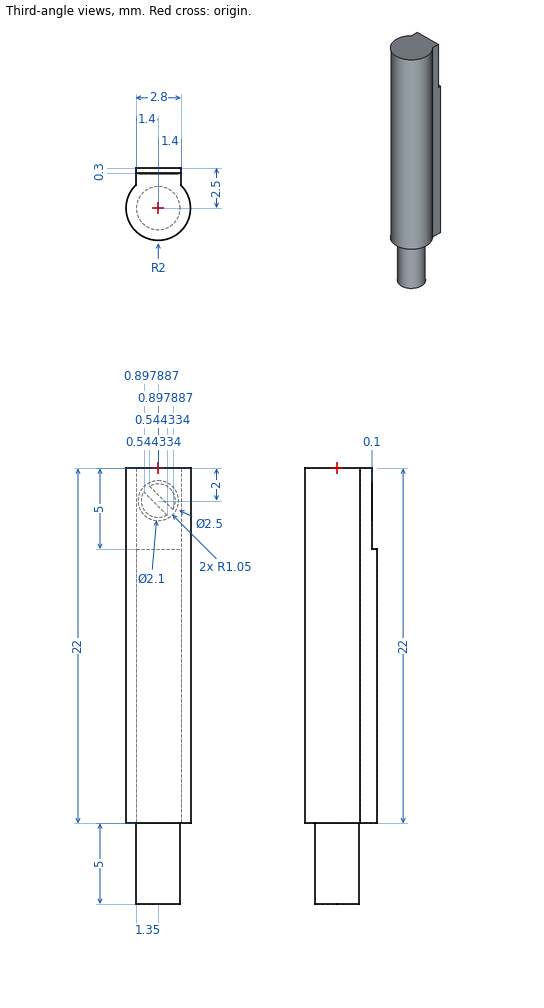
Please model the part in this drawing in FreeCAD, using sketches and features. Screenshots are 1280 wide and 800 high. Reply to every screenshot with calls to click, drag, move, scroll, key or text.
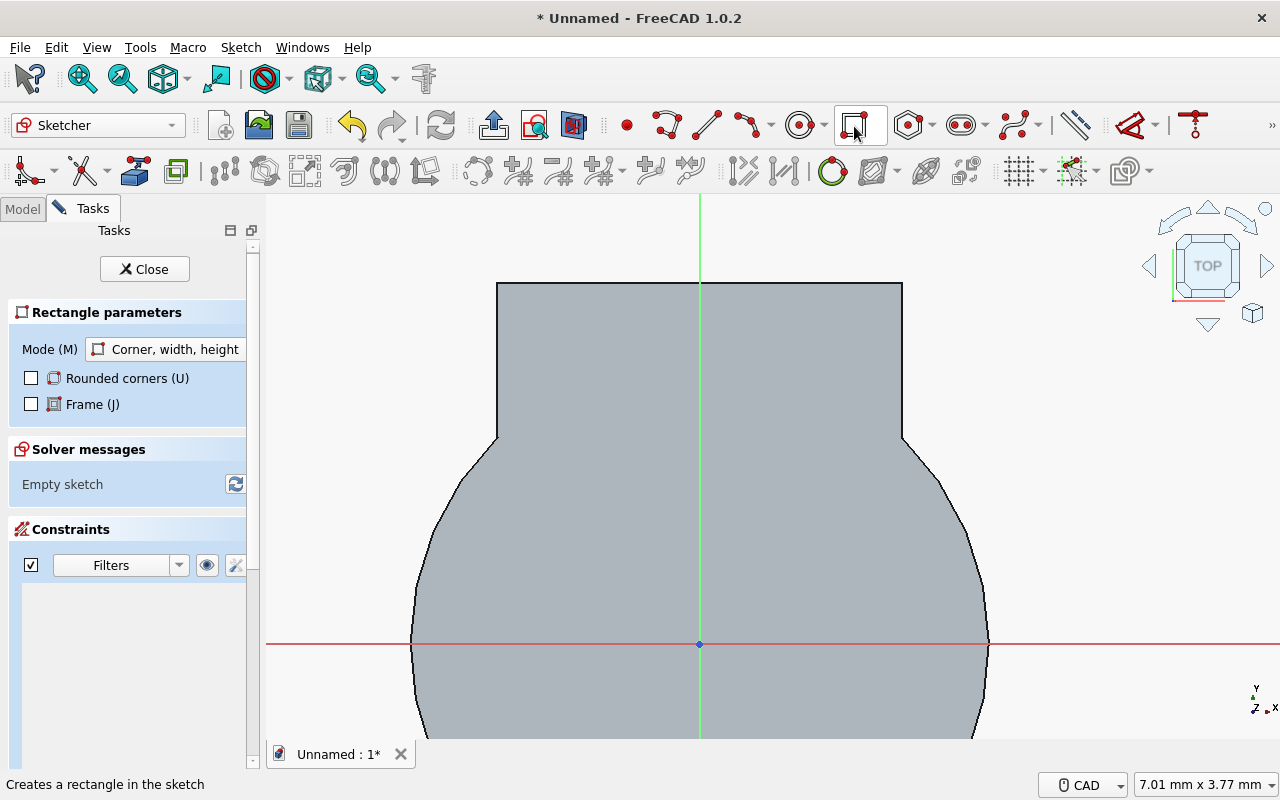
click(497, 283)
click(902, 326)
key(Escape)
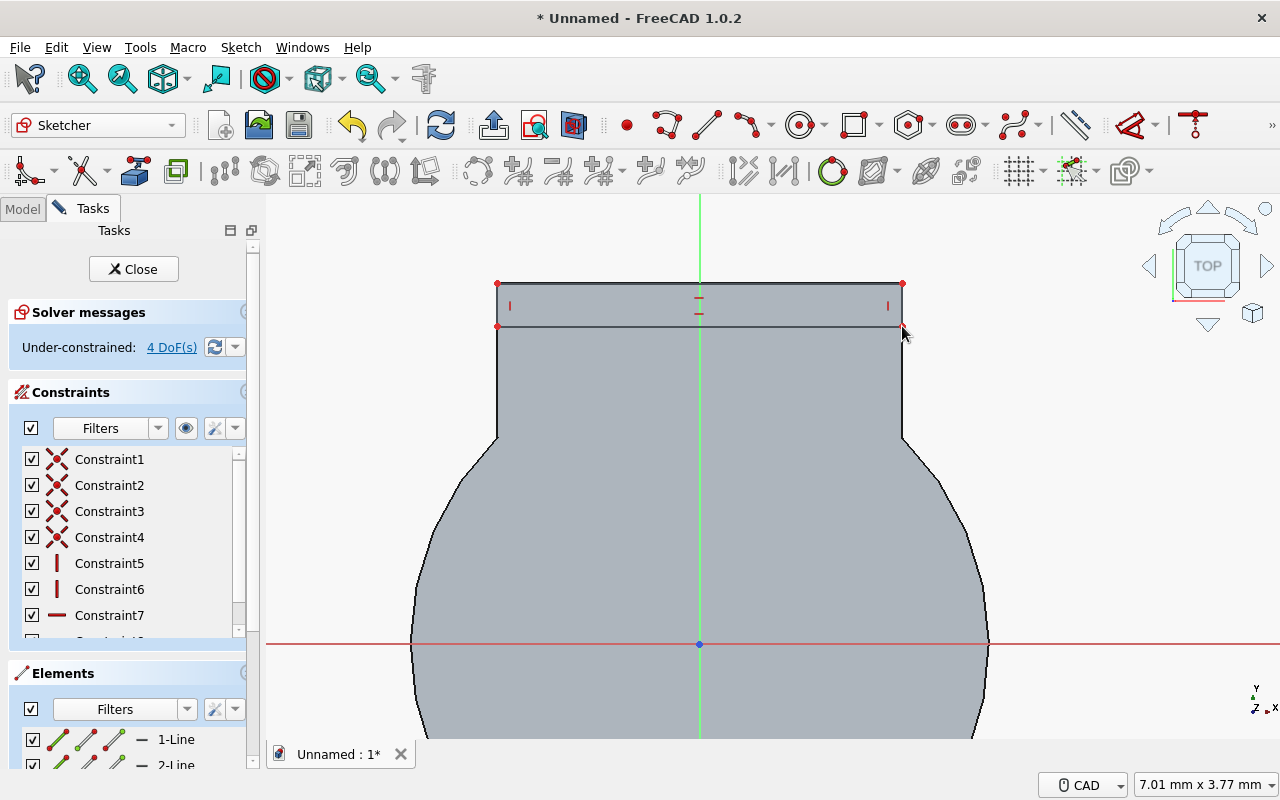
click(1130, 126)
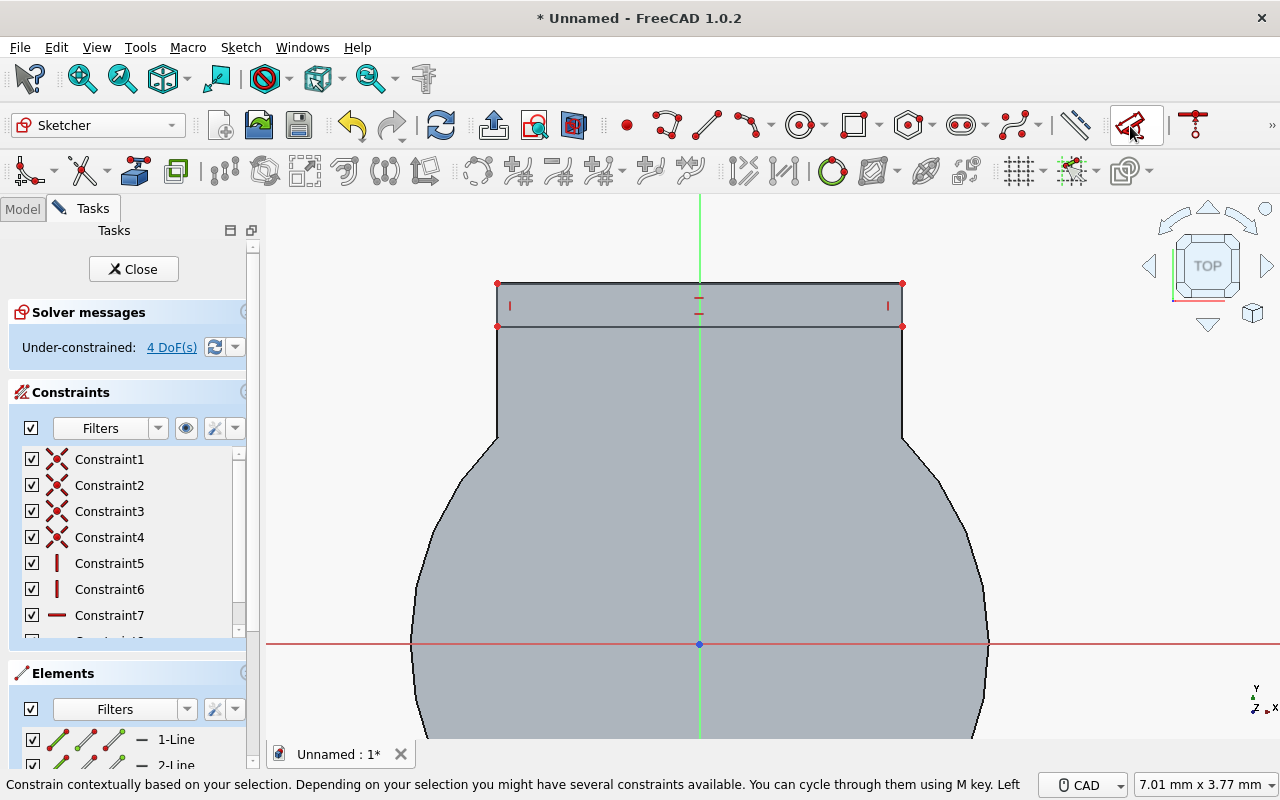
click(497, 297)
click(463, 305)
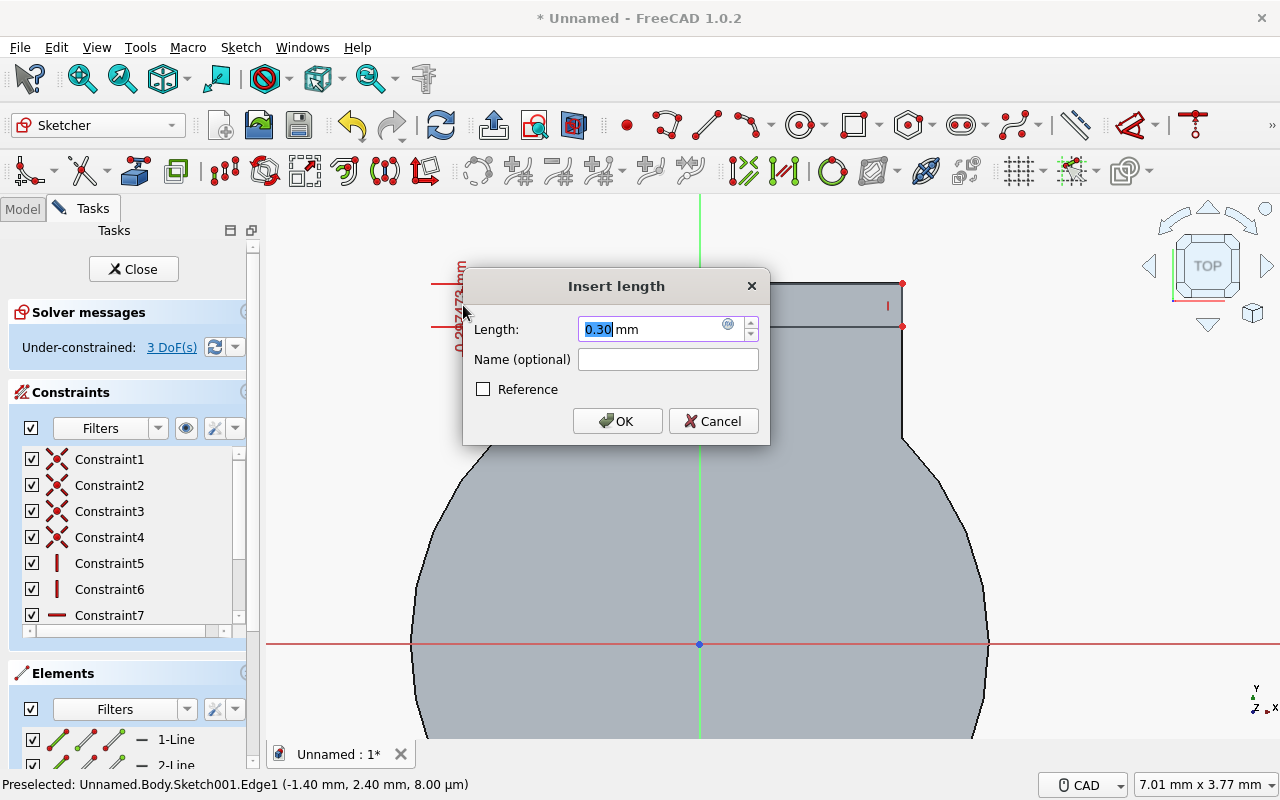
text(0.3)
key(Return)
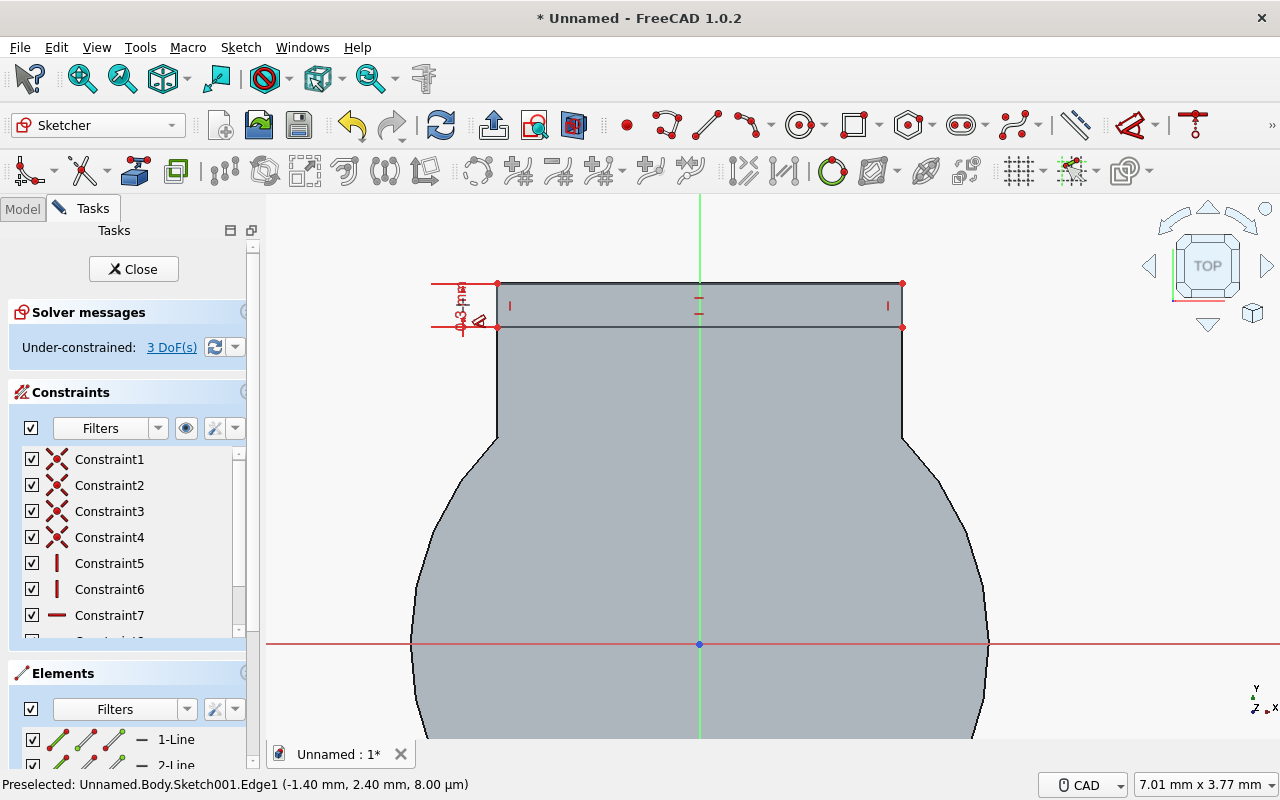
click(619, 327)
click(606, 361)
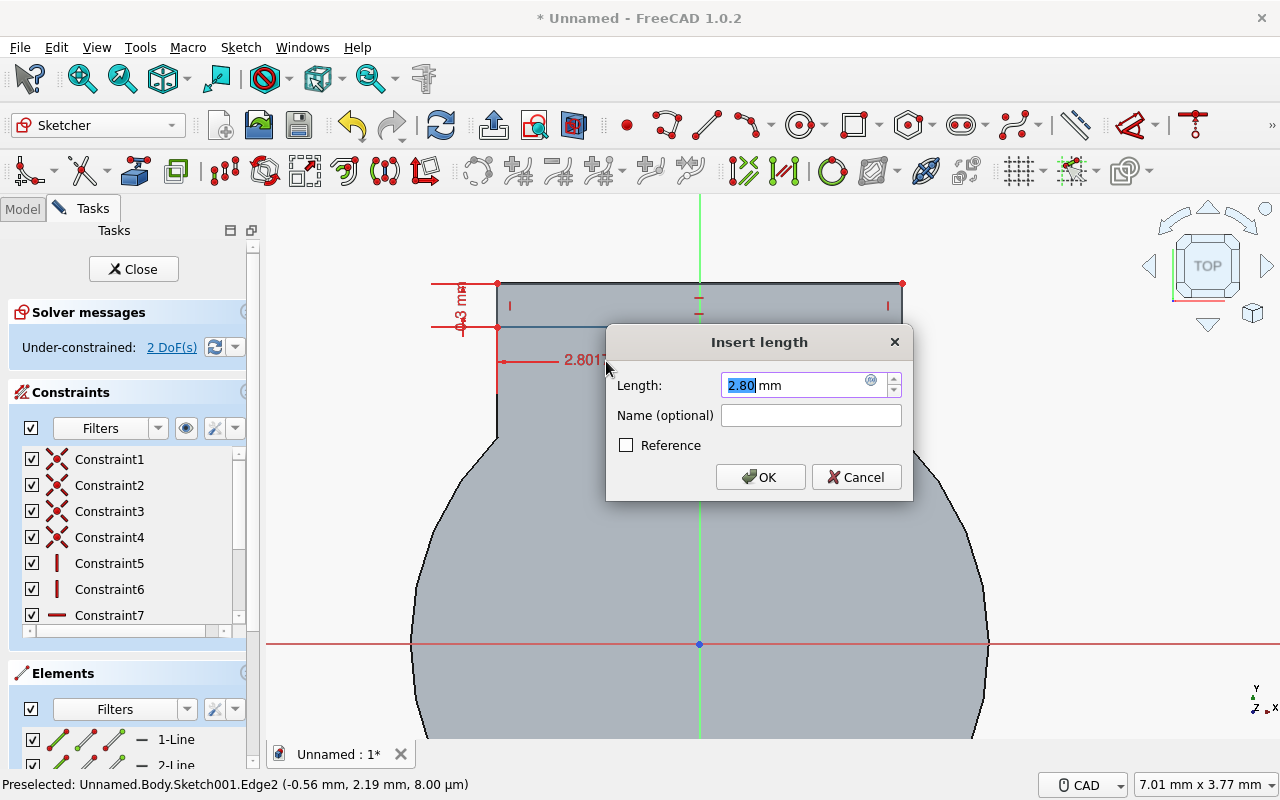
text(2.8)
key(Return)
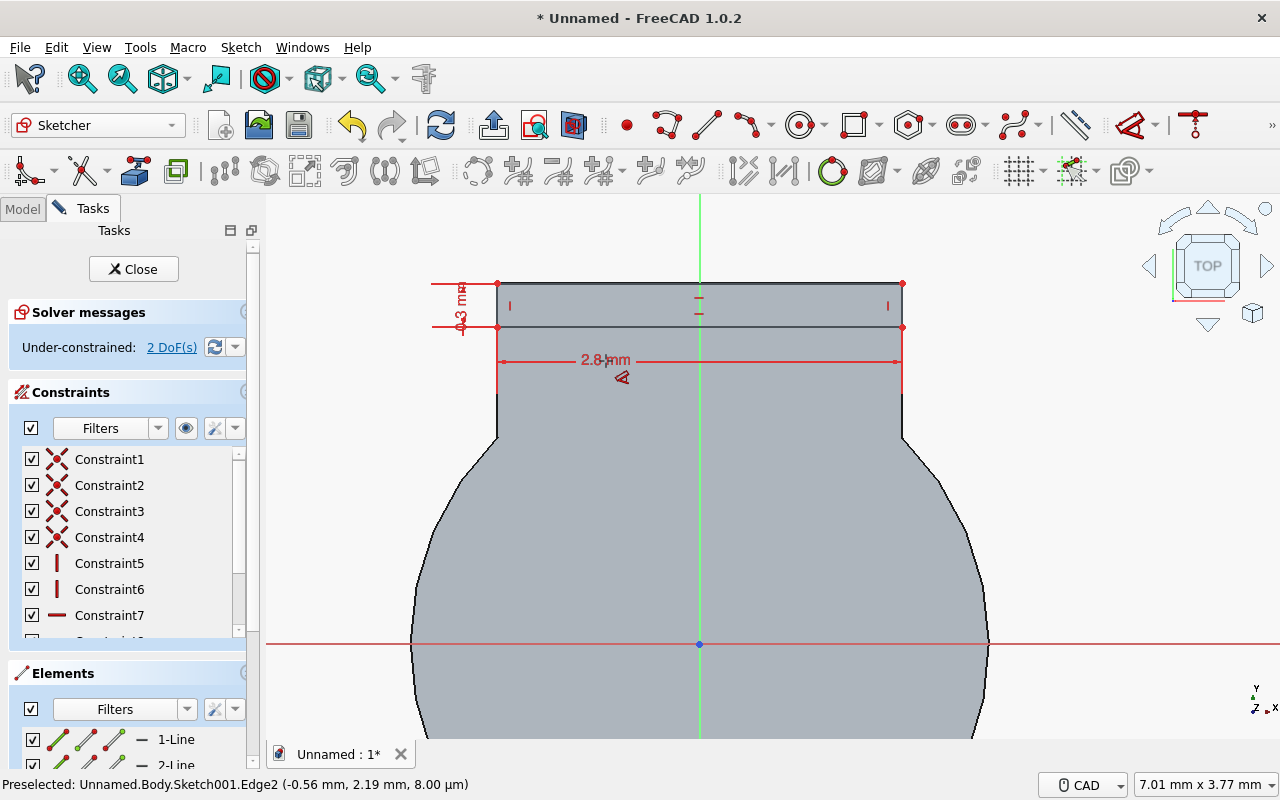
click(497, 284)
click(598, 678)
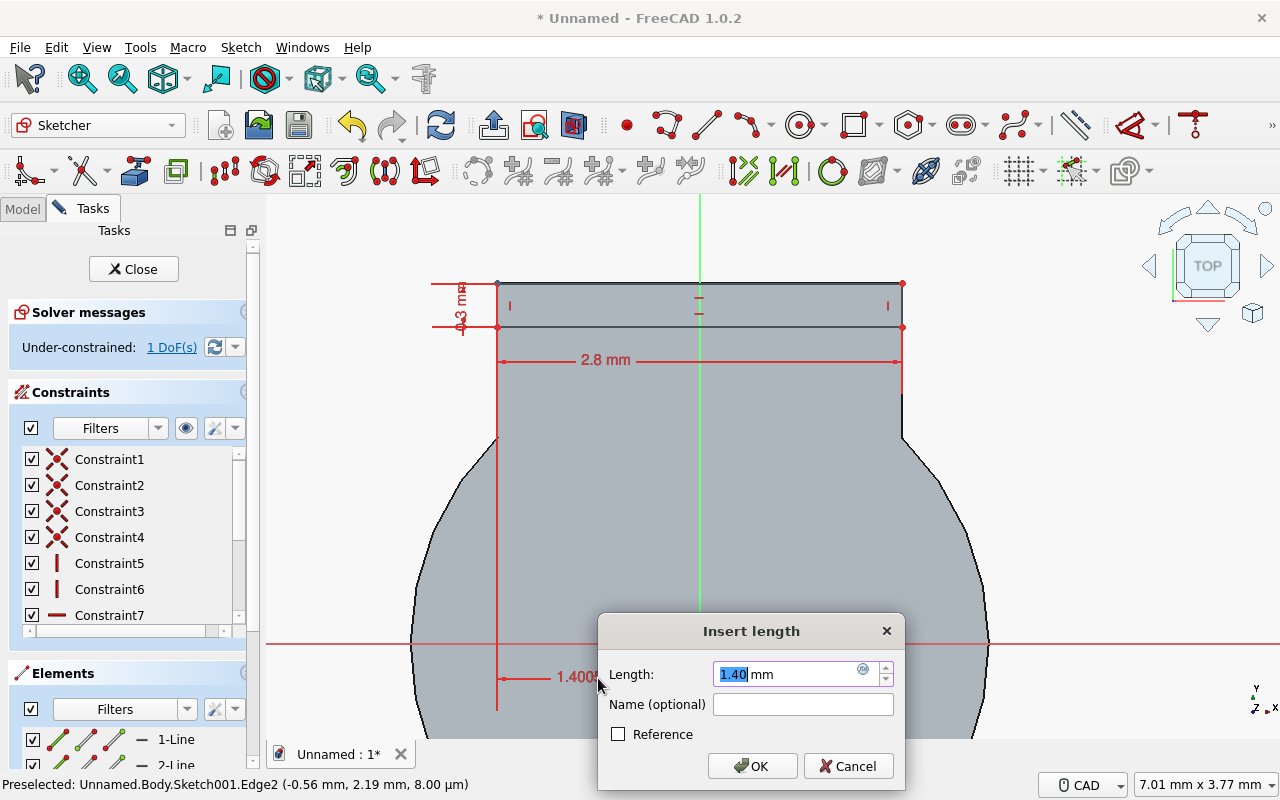
text(1.4)
key(Return)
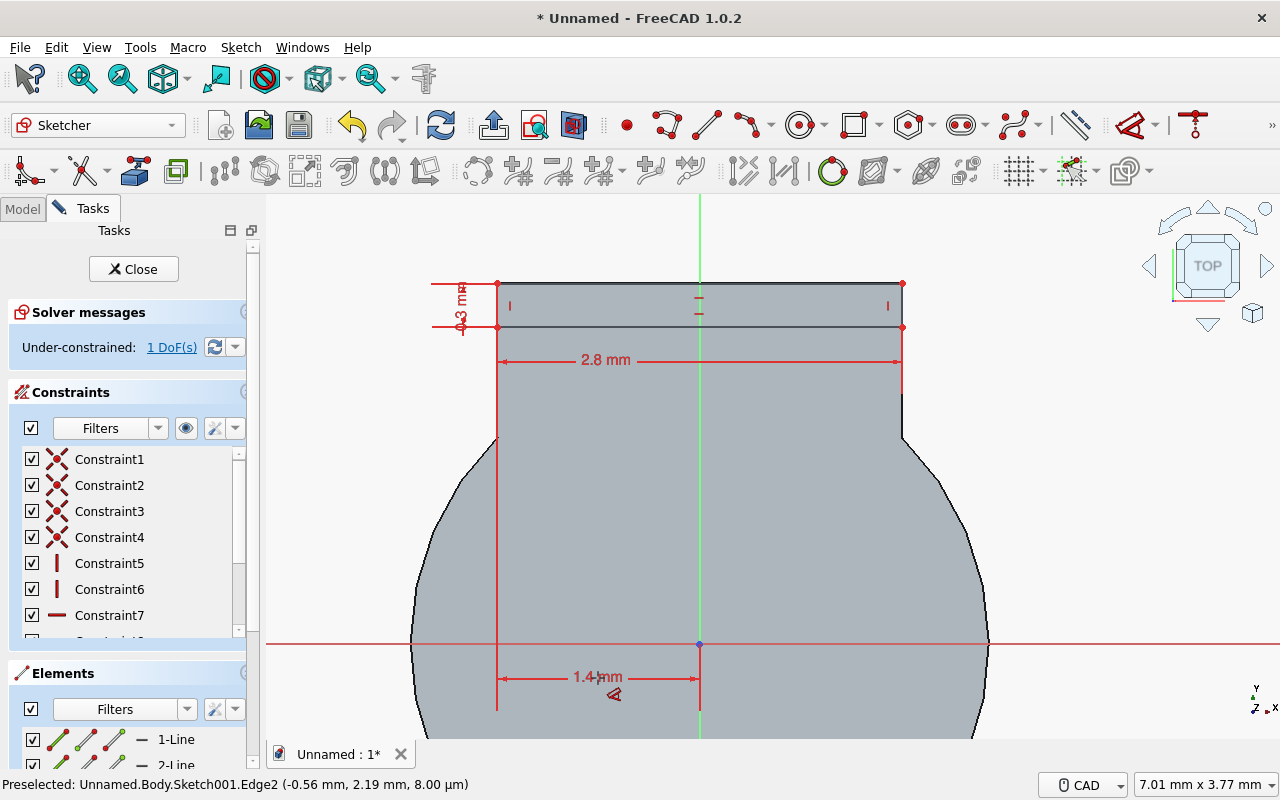
click(497, 284)
click(463, 464)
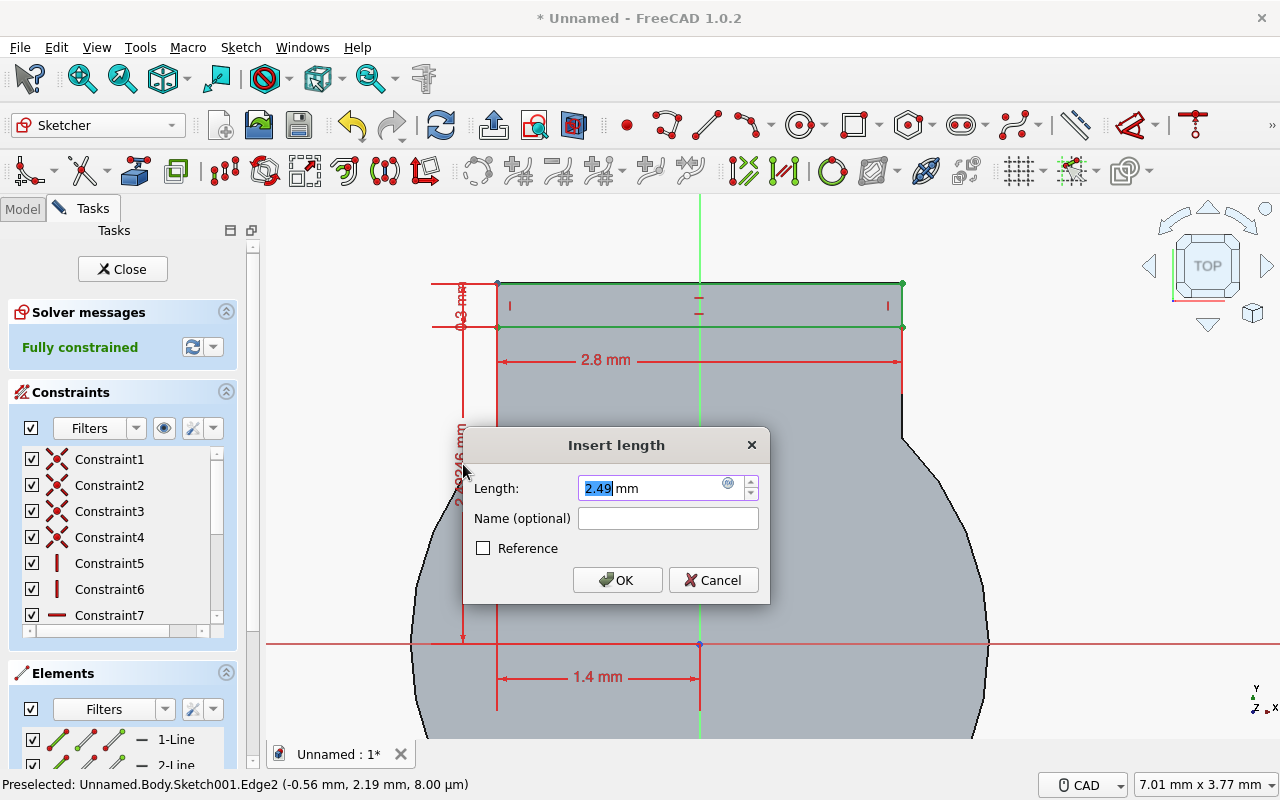
text(2.5)
key(Return)
key(Escape)